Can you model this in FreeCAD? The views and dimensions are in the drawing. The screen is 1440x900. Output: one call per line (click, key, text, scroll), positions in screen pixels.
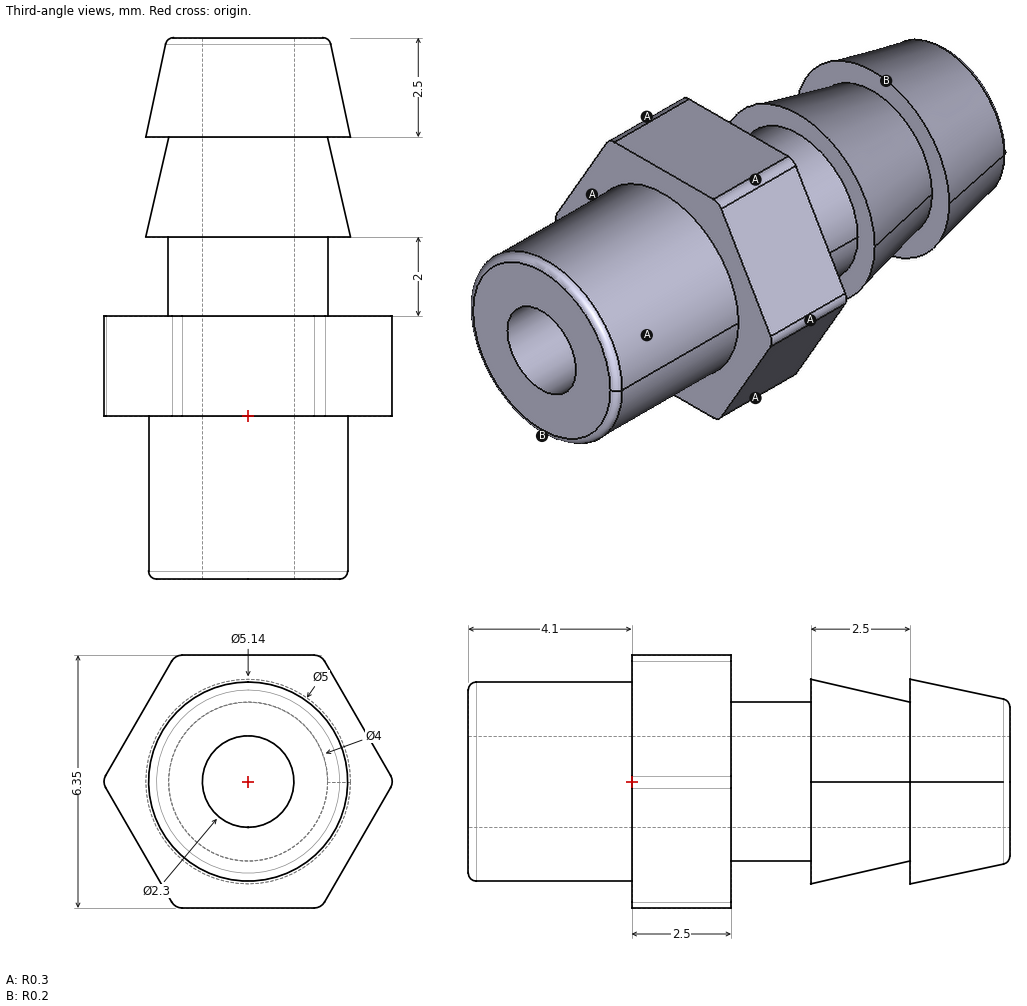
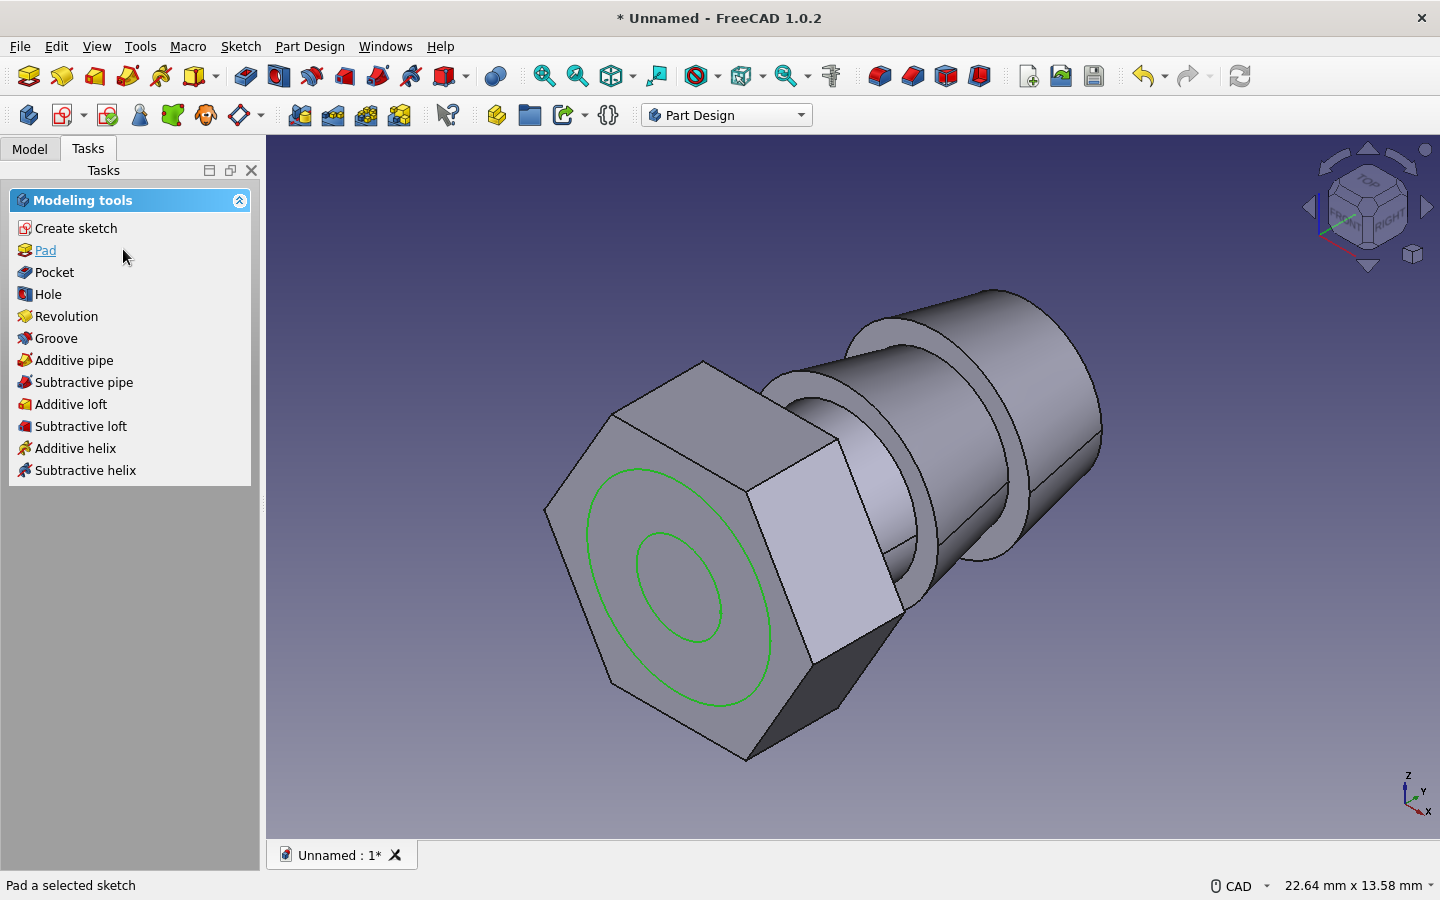
click(29, 76)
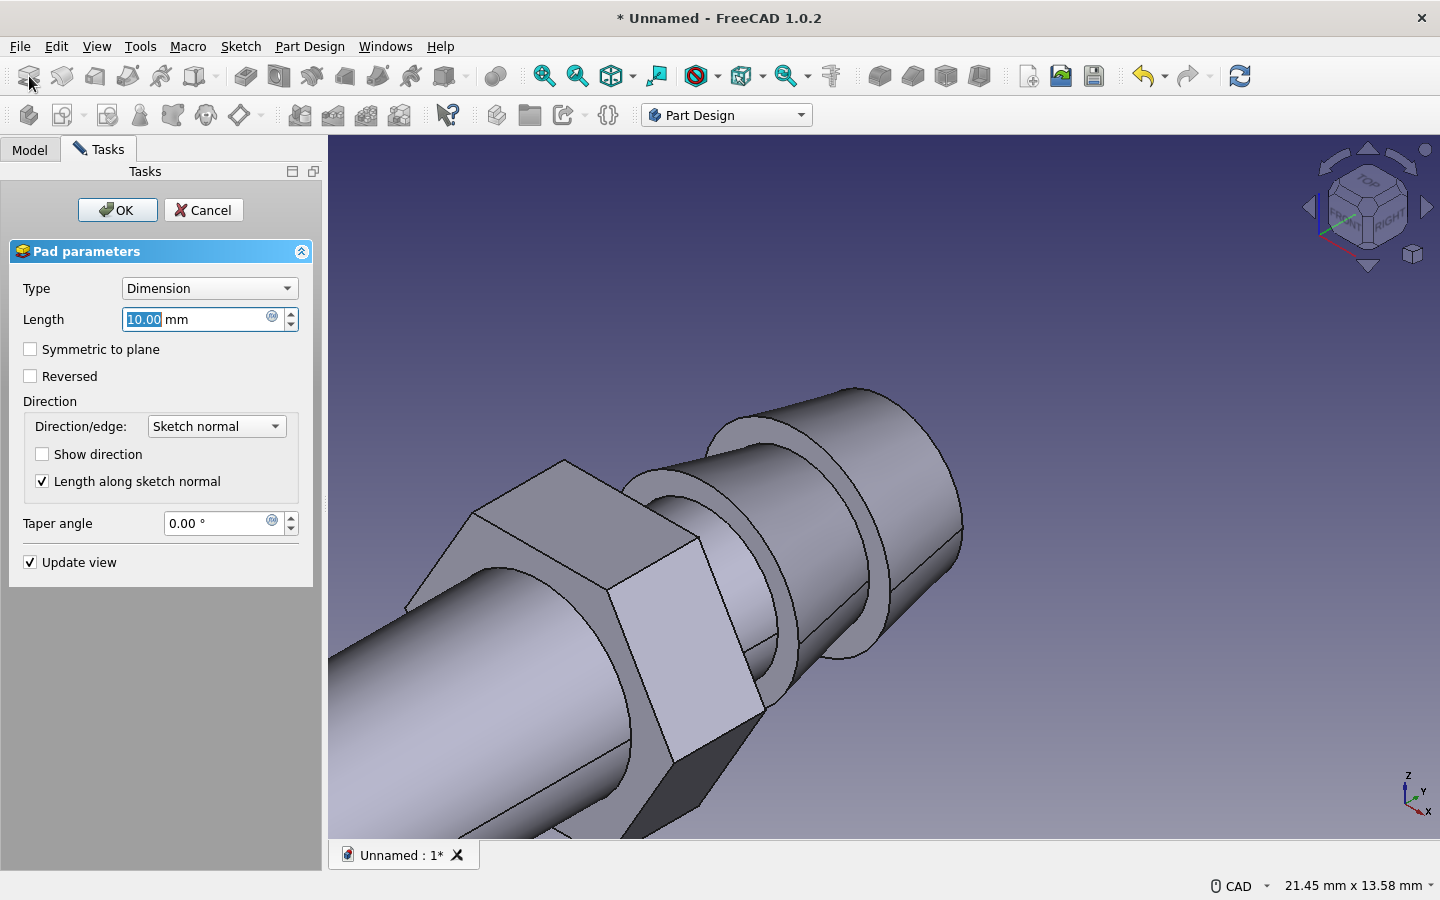
text(4.1)
key(Tab)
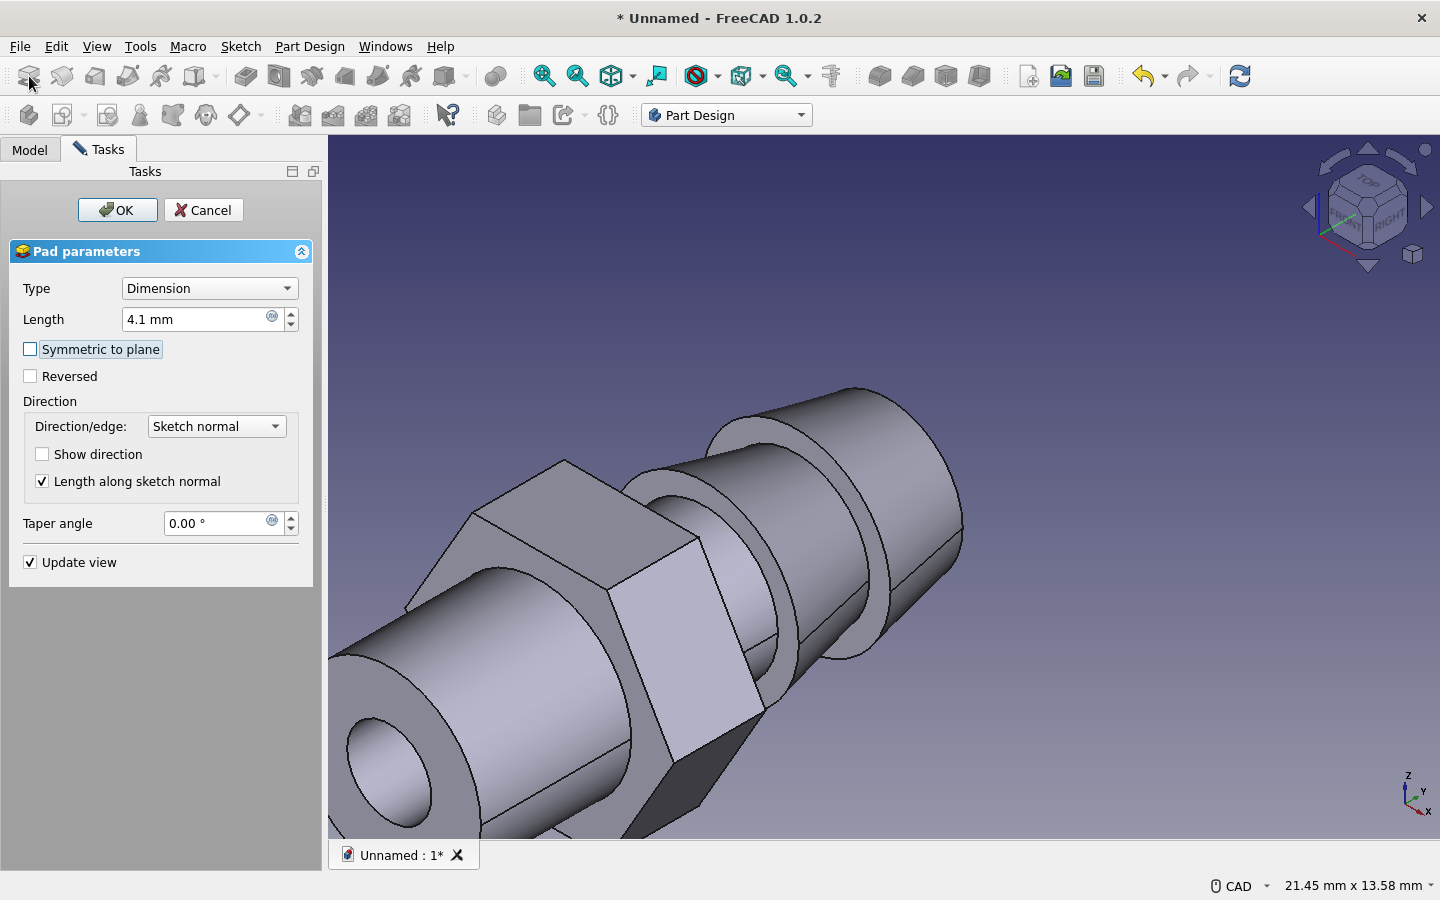
click(118, 210)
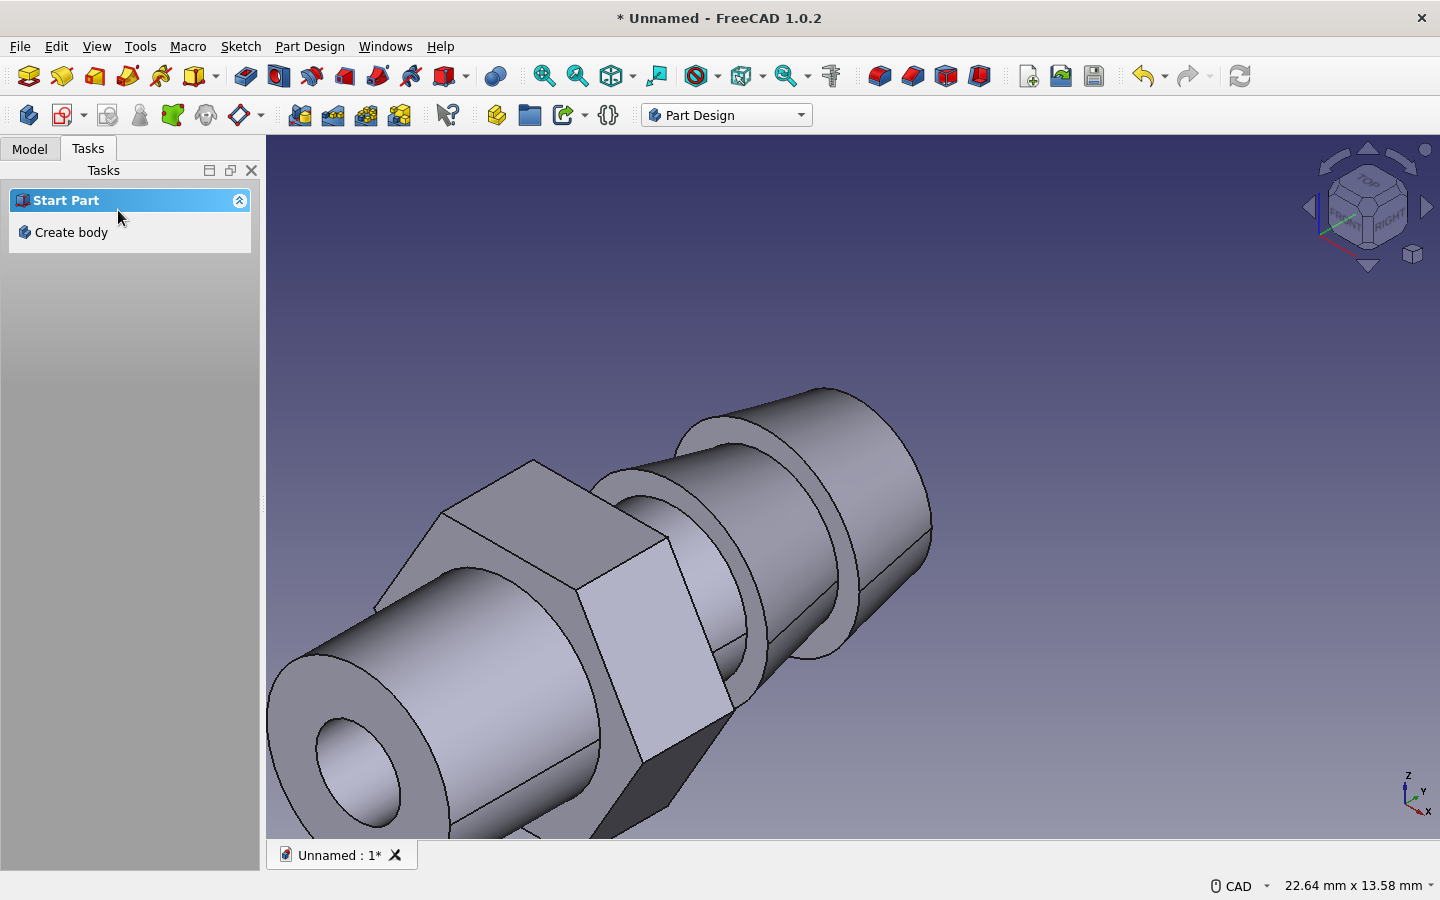
click(545, 76)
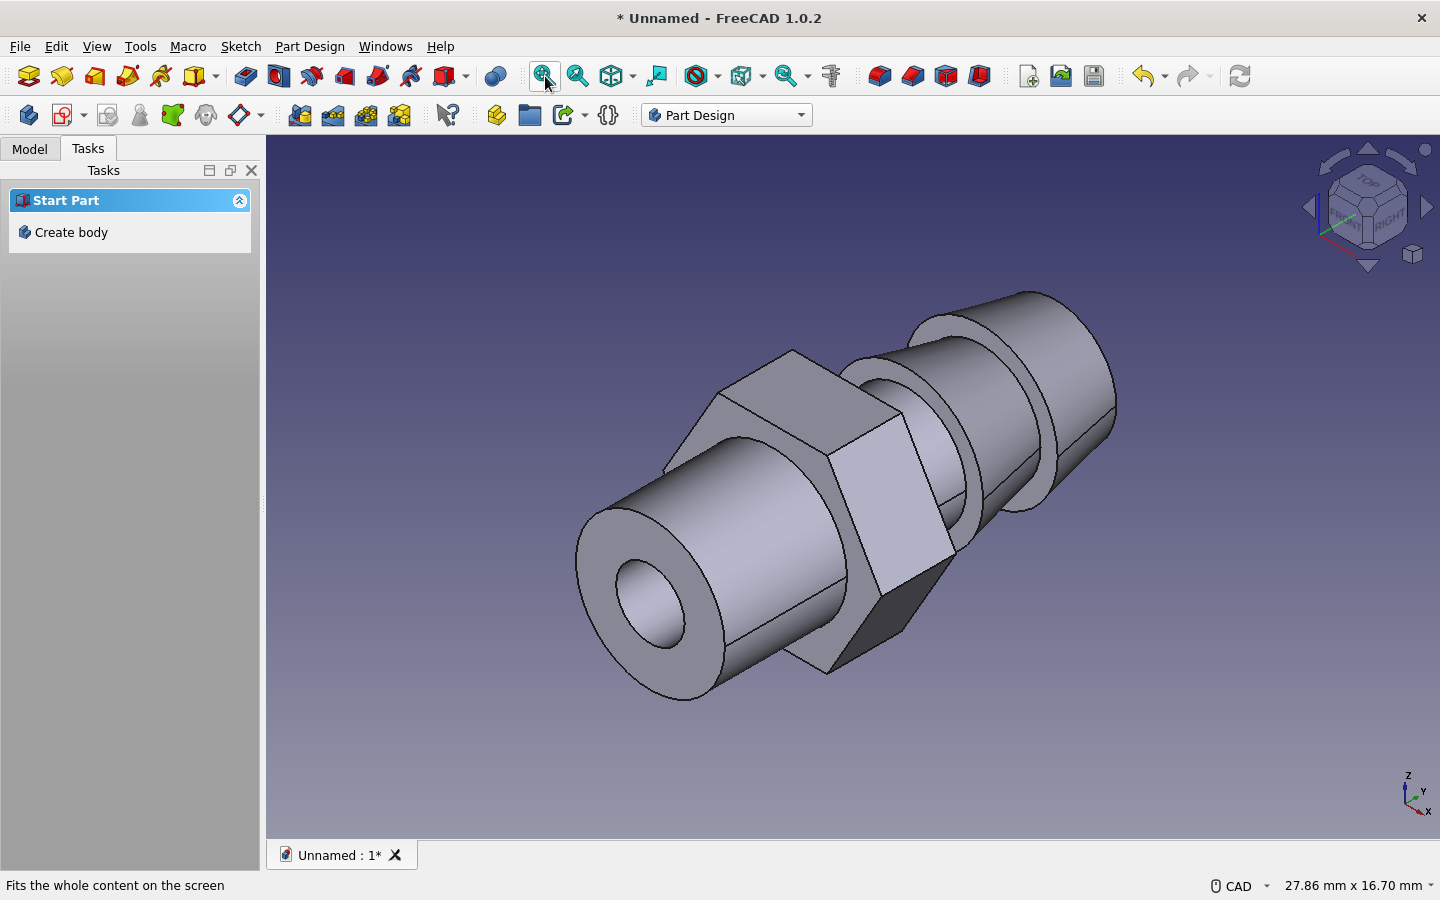
click(62, 116)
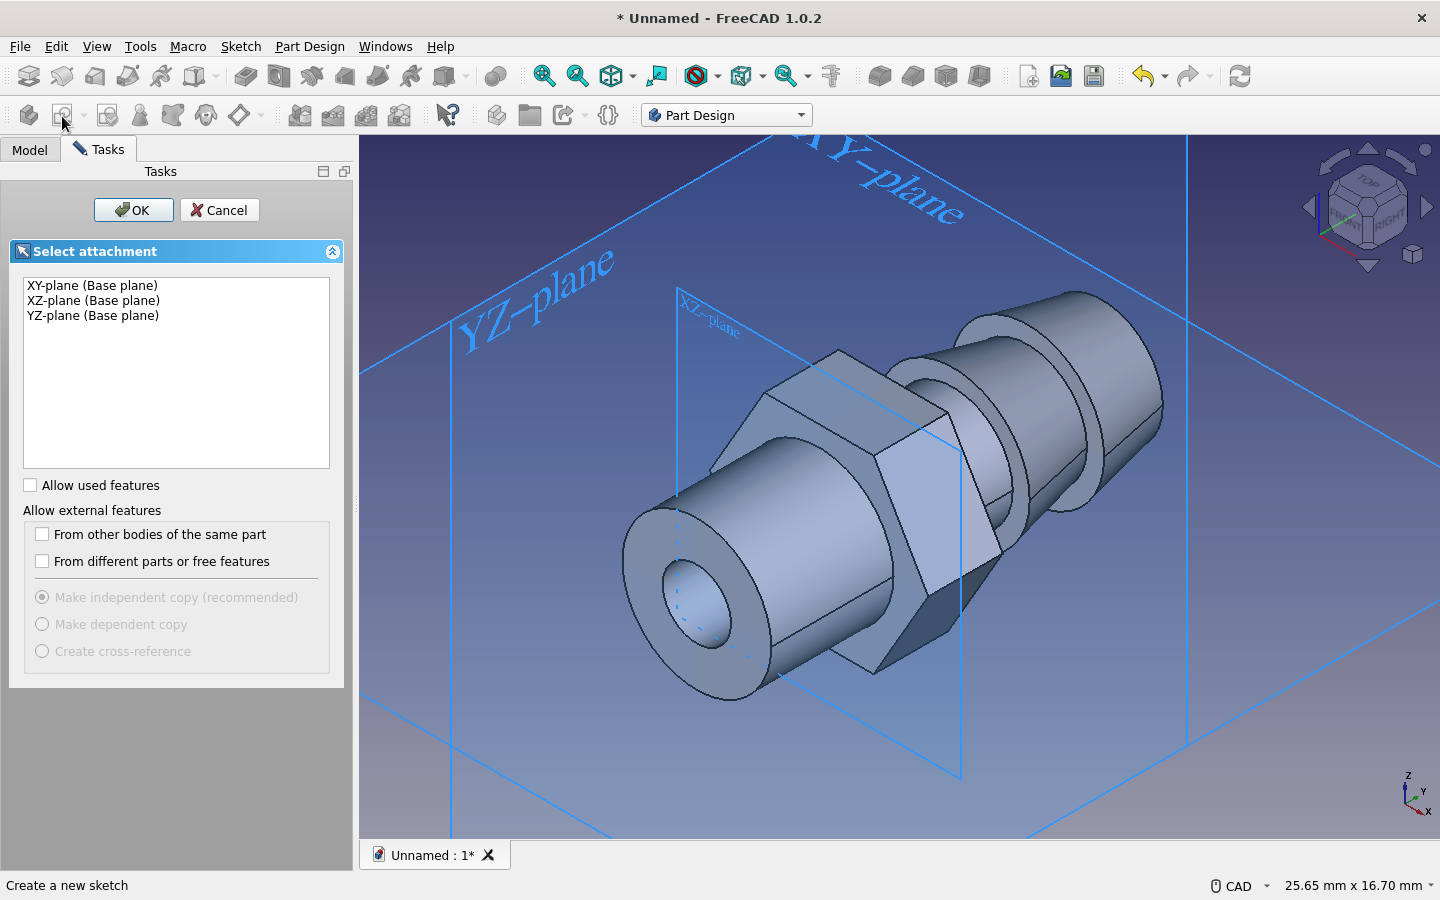
click(84, 300)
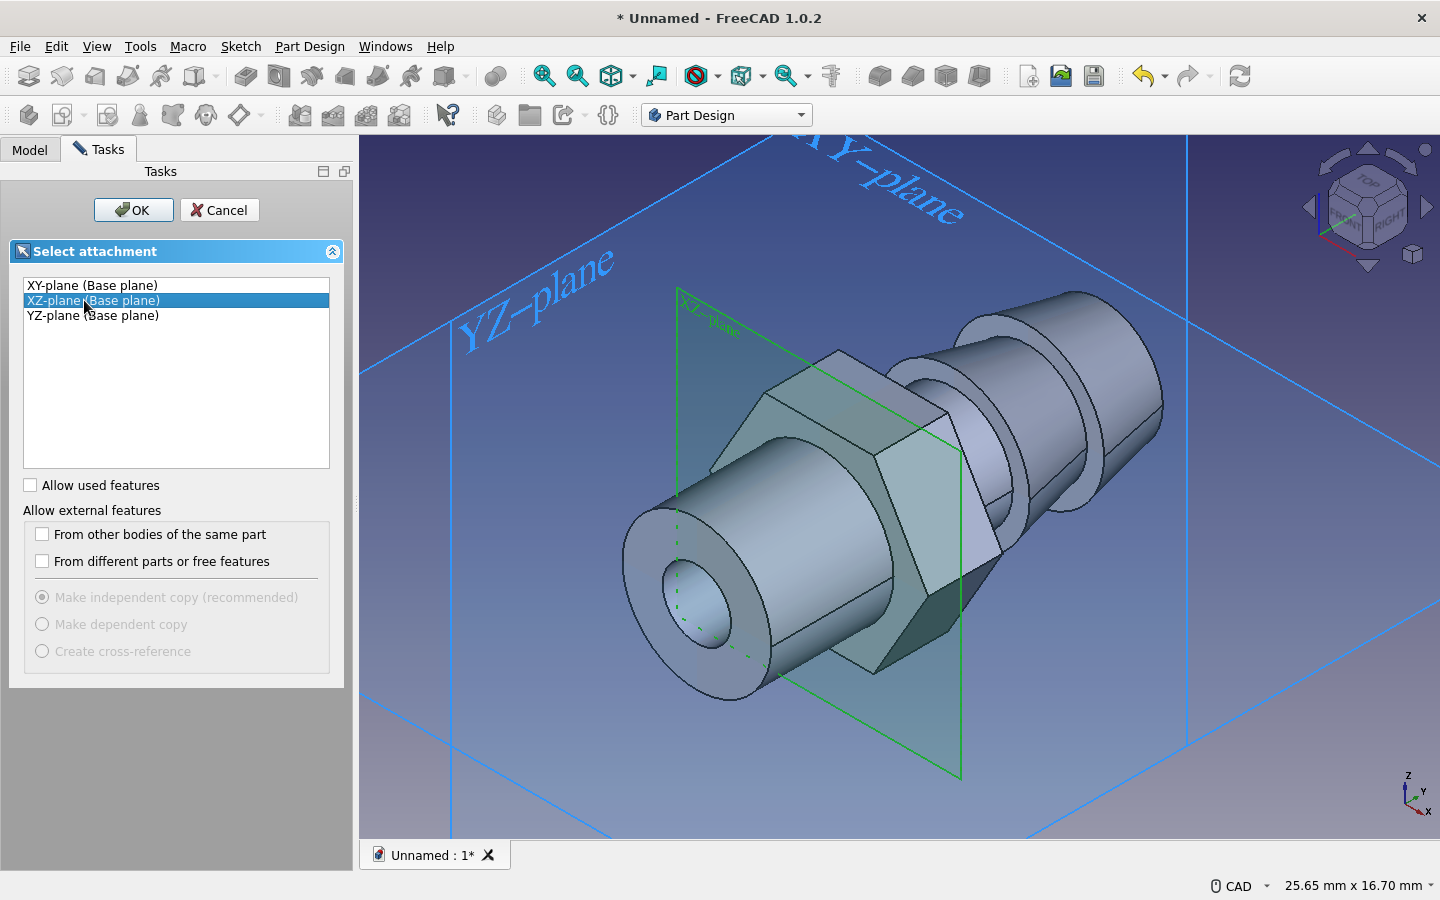
click(134, 210)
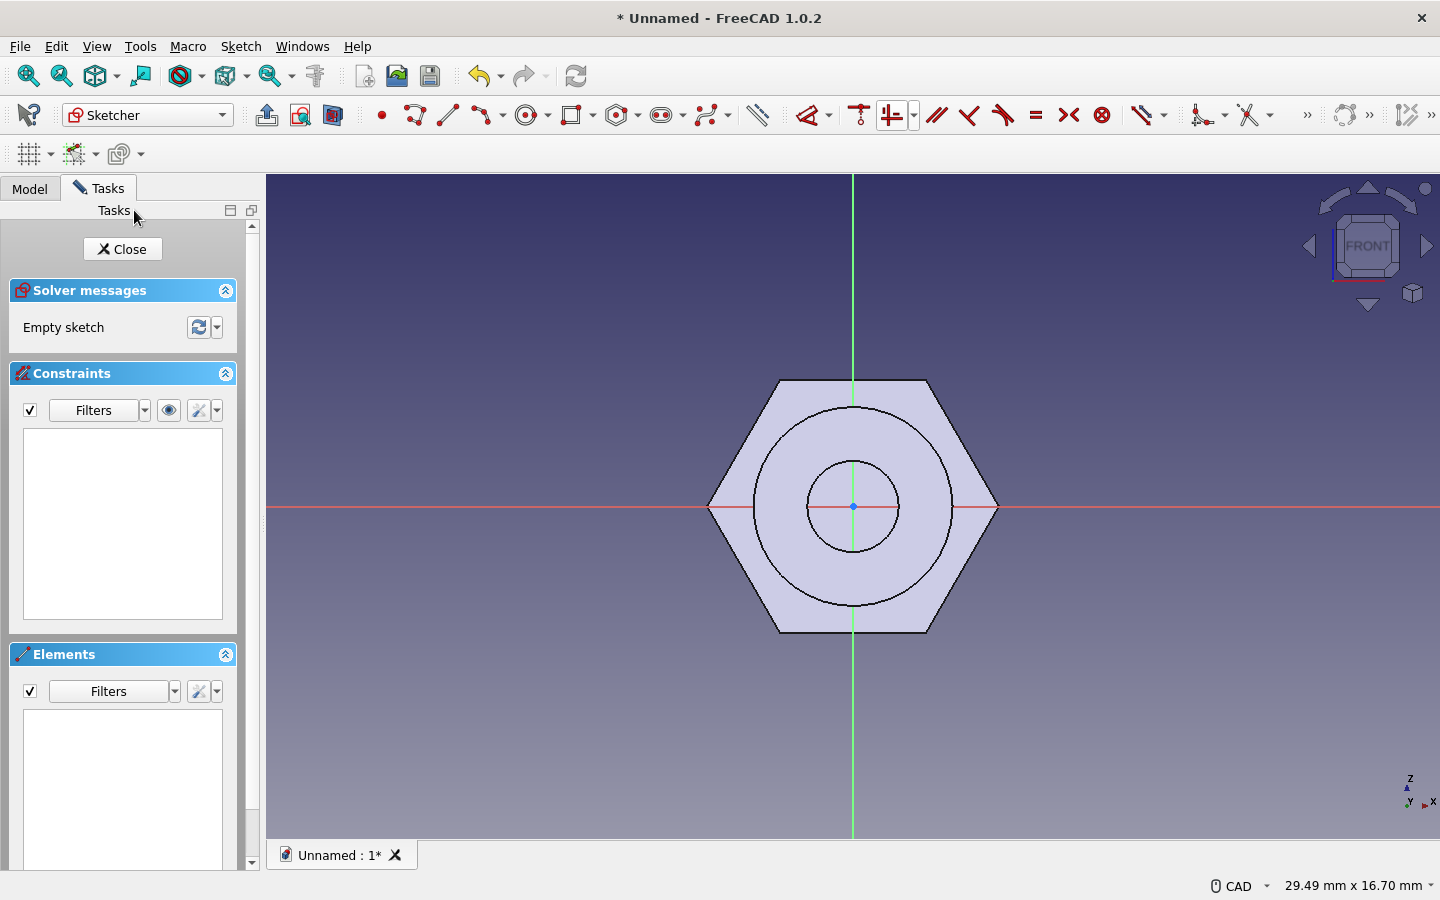
click(333, 116)